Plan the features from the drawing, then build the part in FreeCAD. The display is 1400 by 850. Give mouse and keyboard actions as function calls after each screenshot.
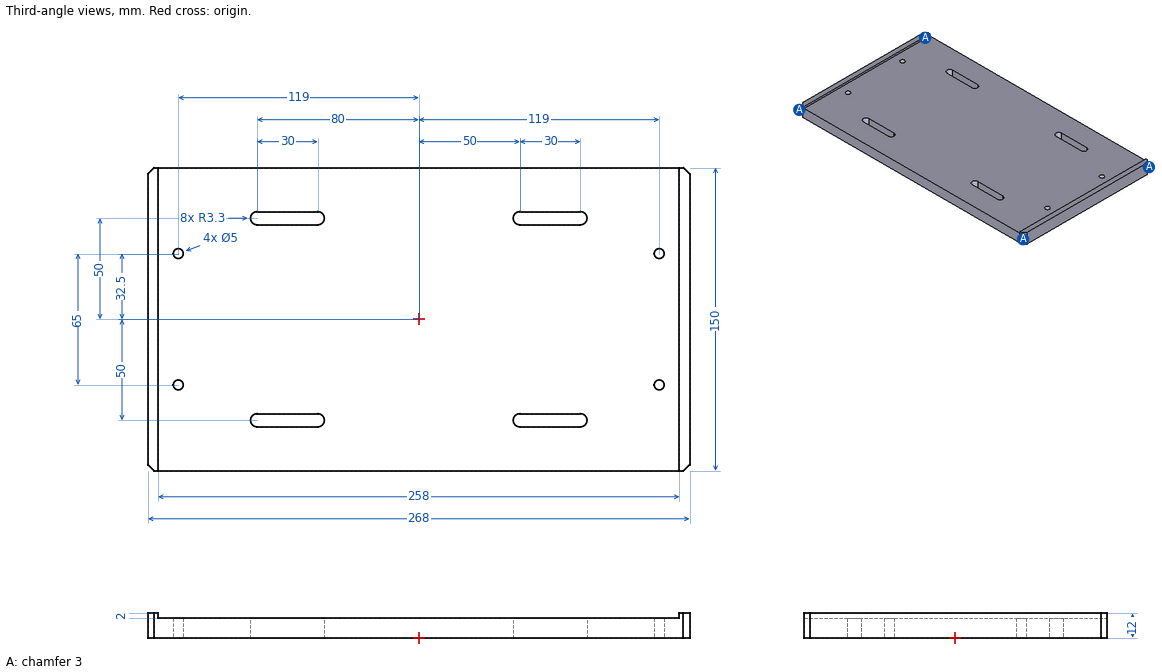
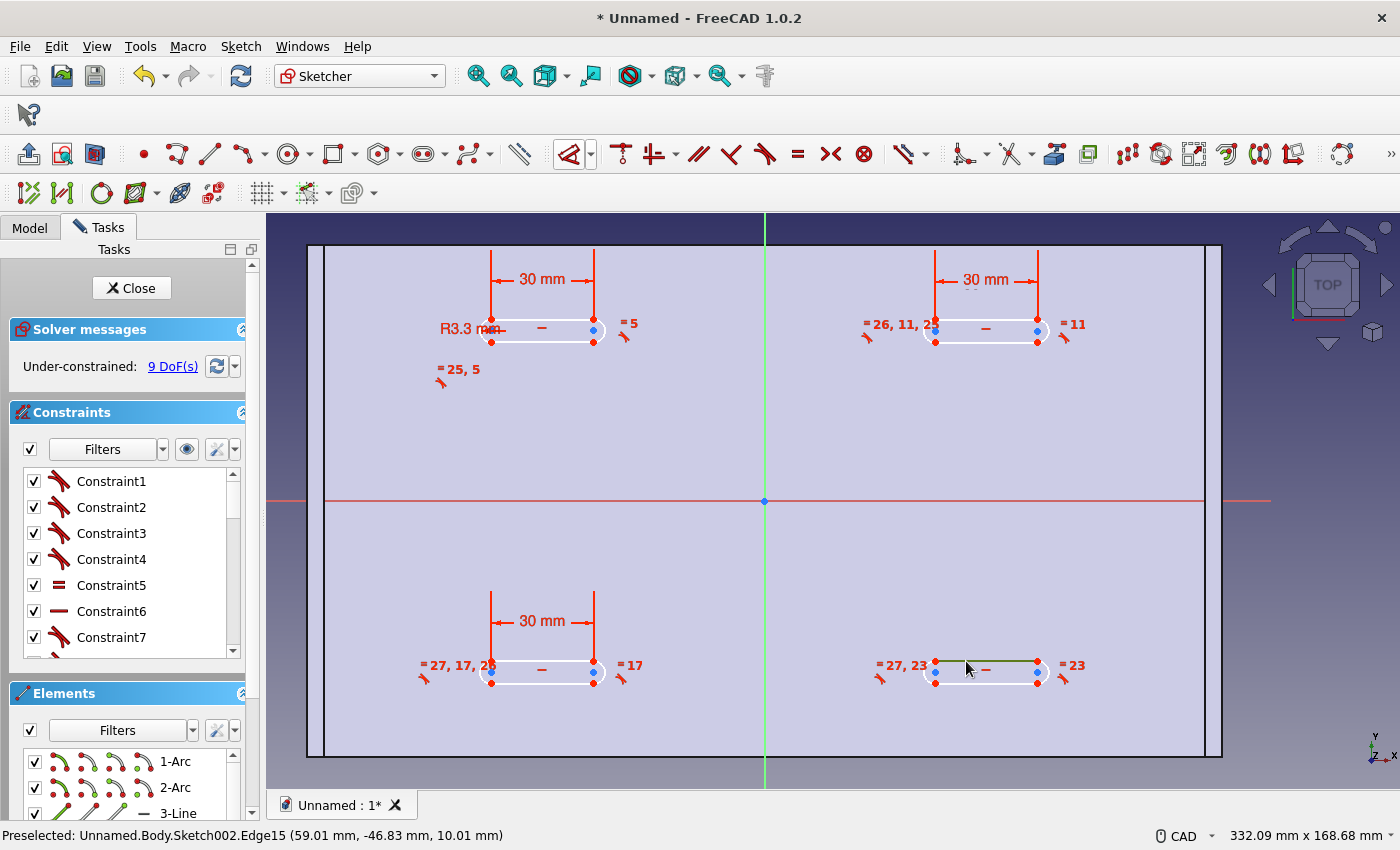
click(590, 154)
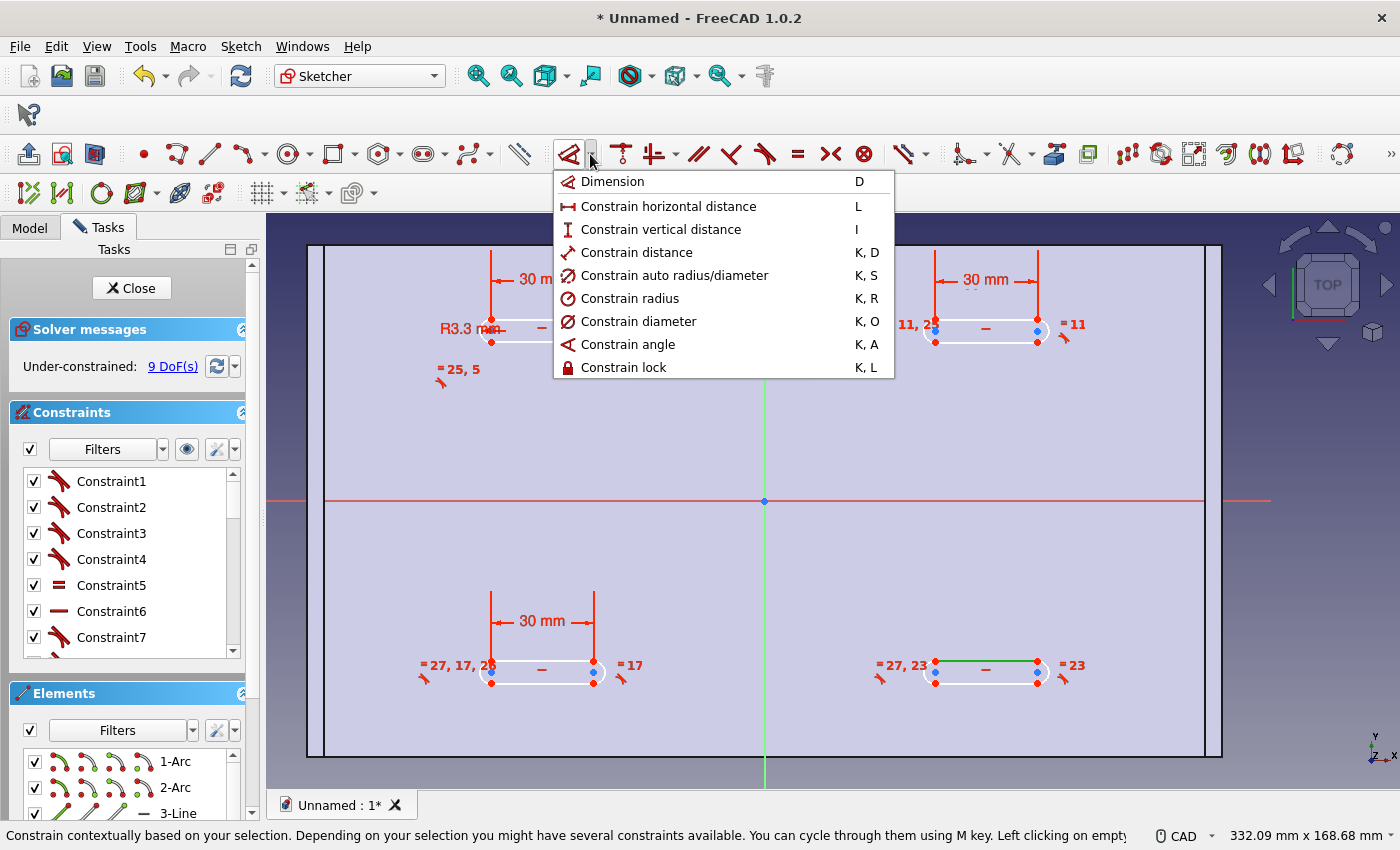
click(724, 206)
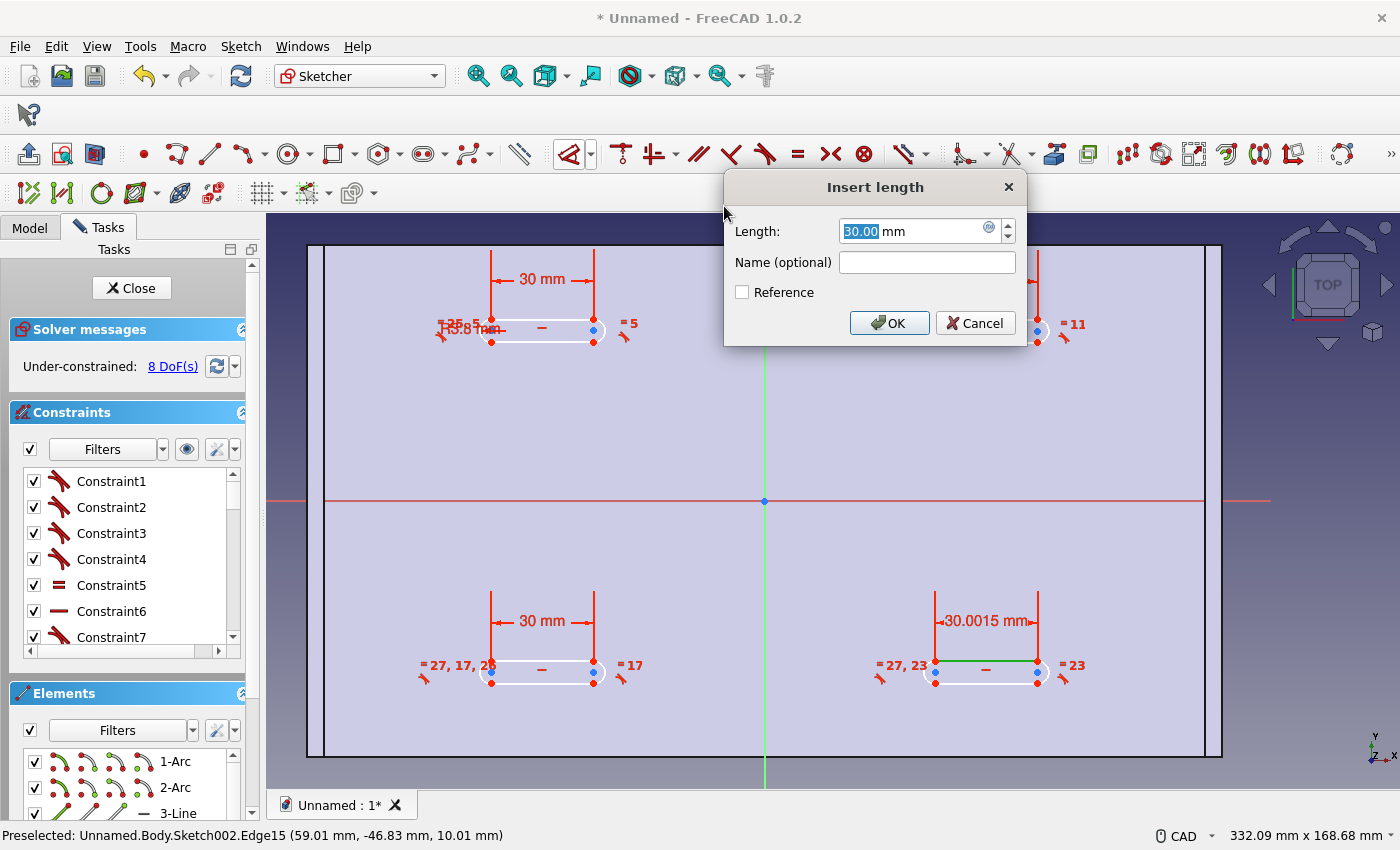
text(30)
key(Return)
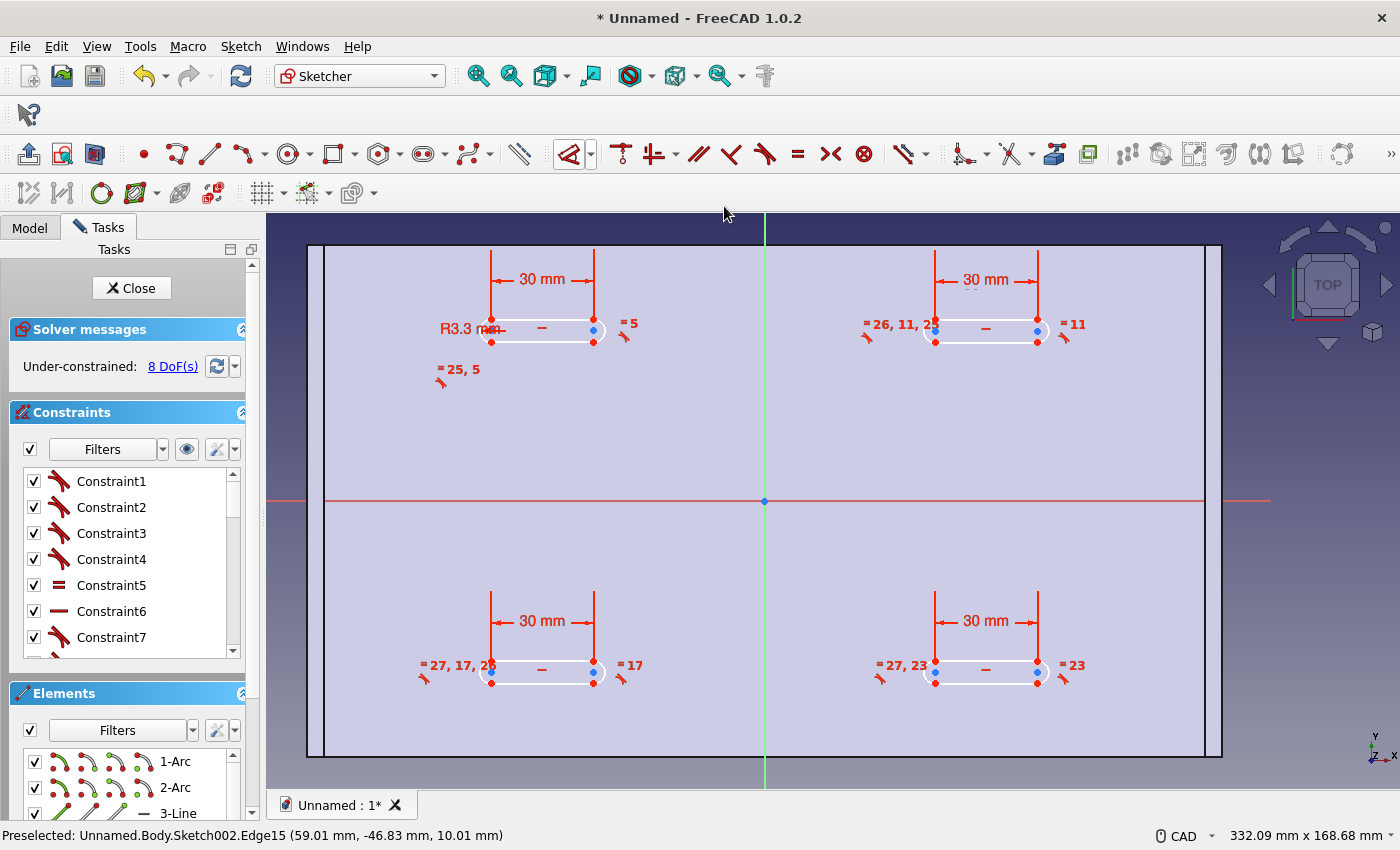
click(491, 320)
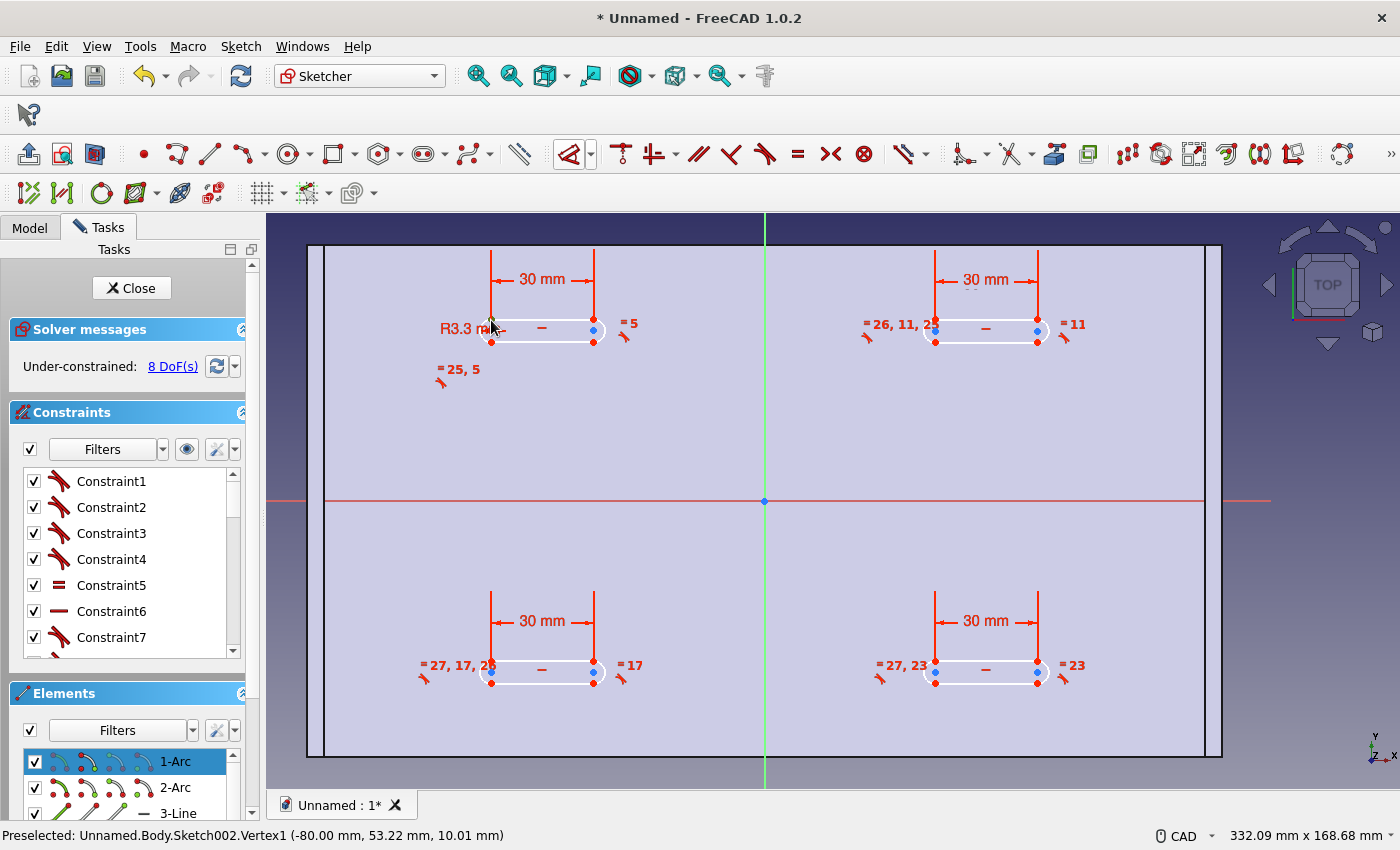
click(590, 154)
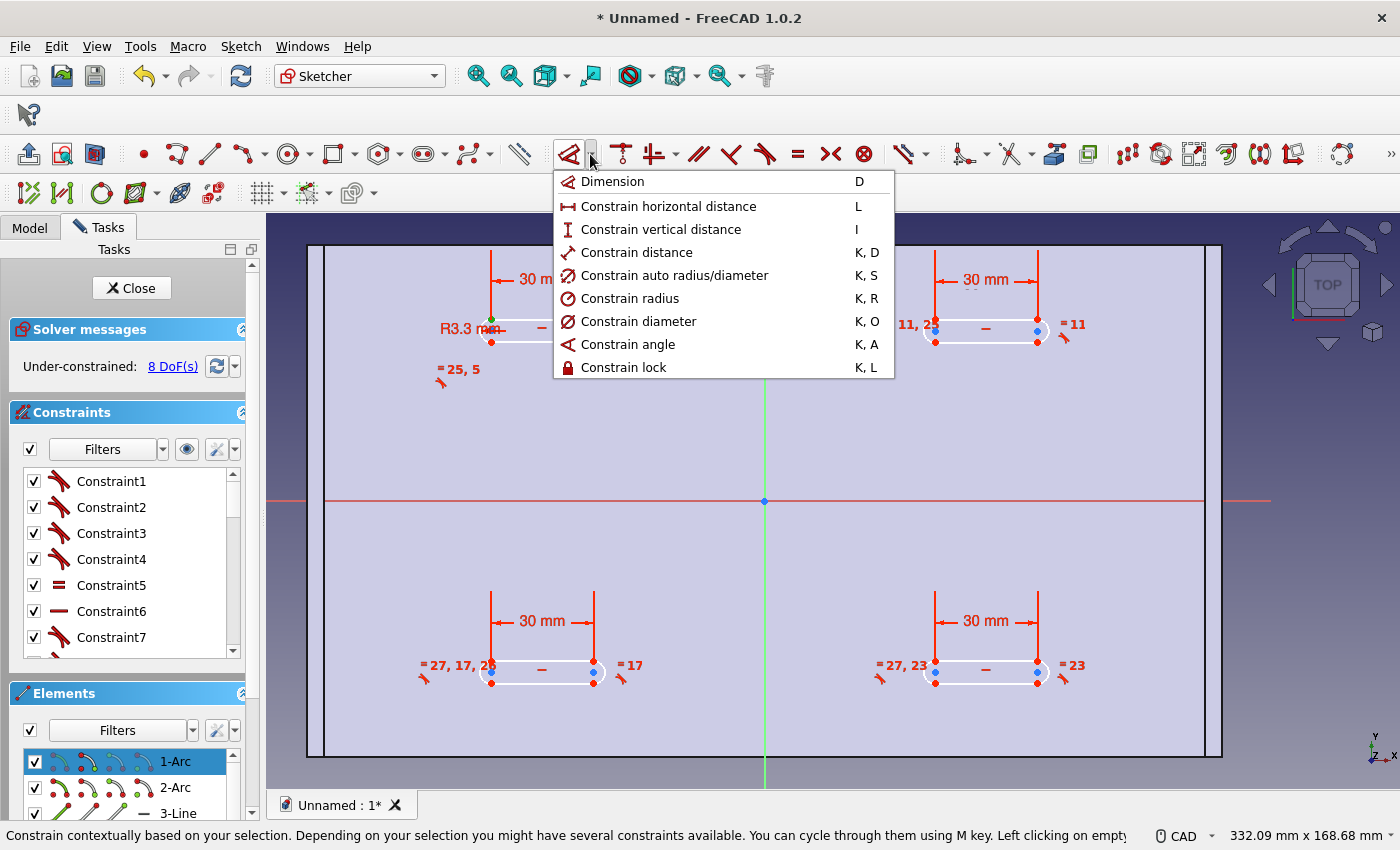
click(724, 206)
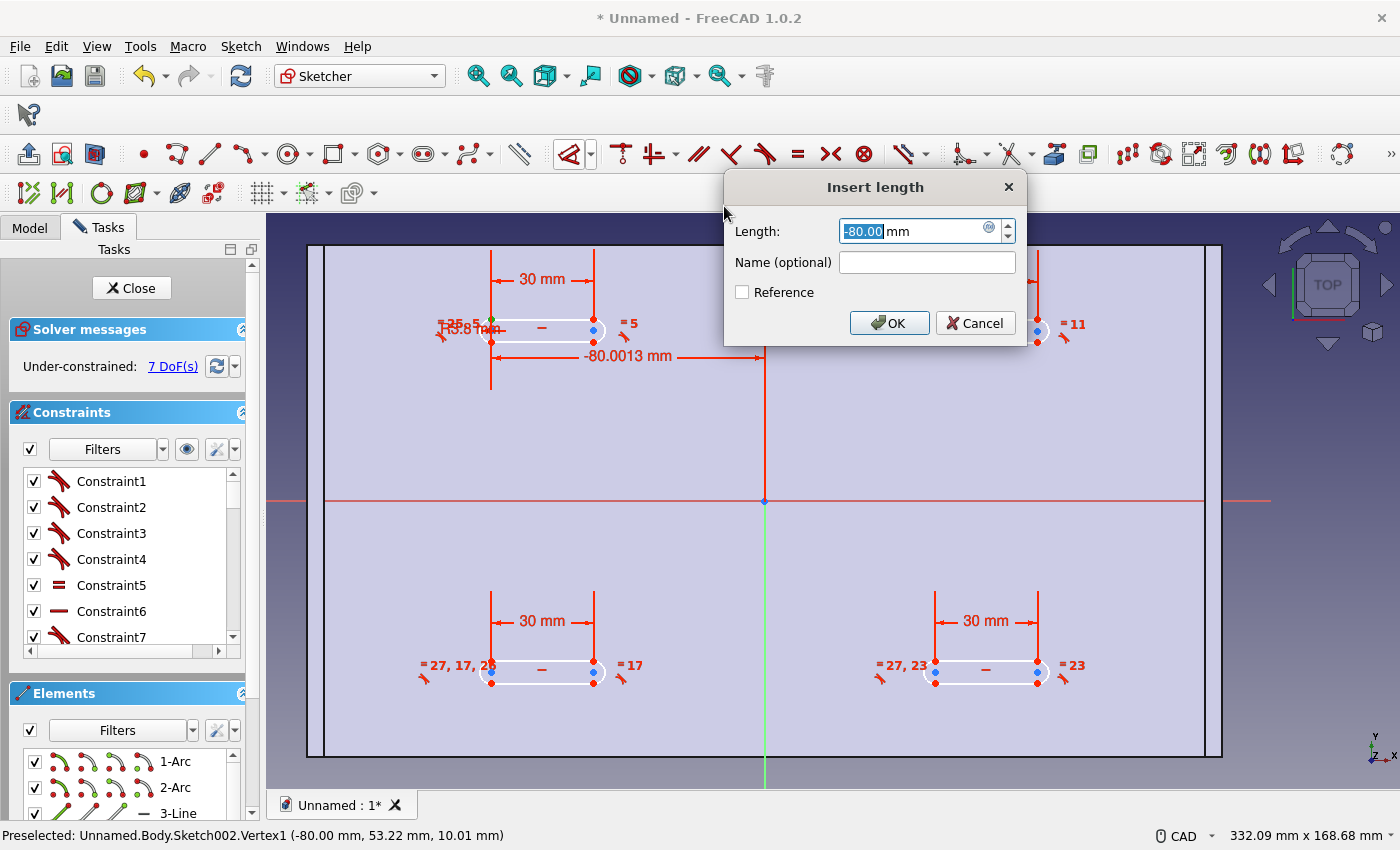
text(-80)
key(Return)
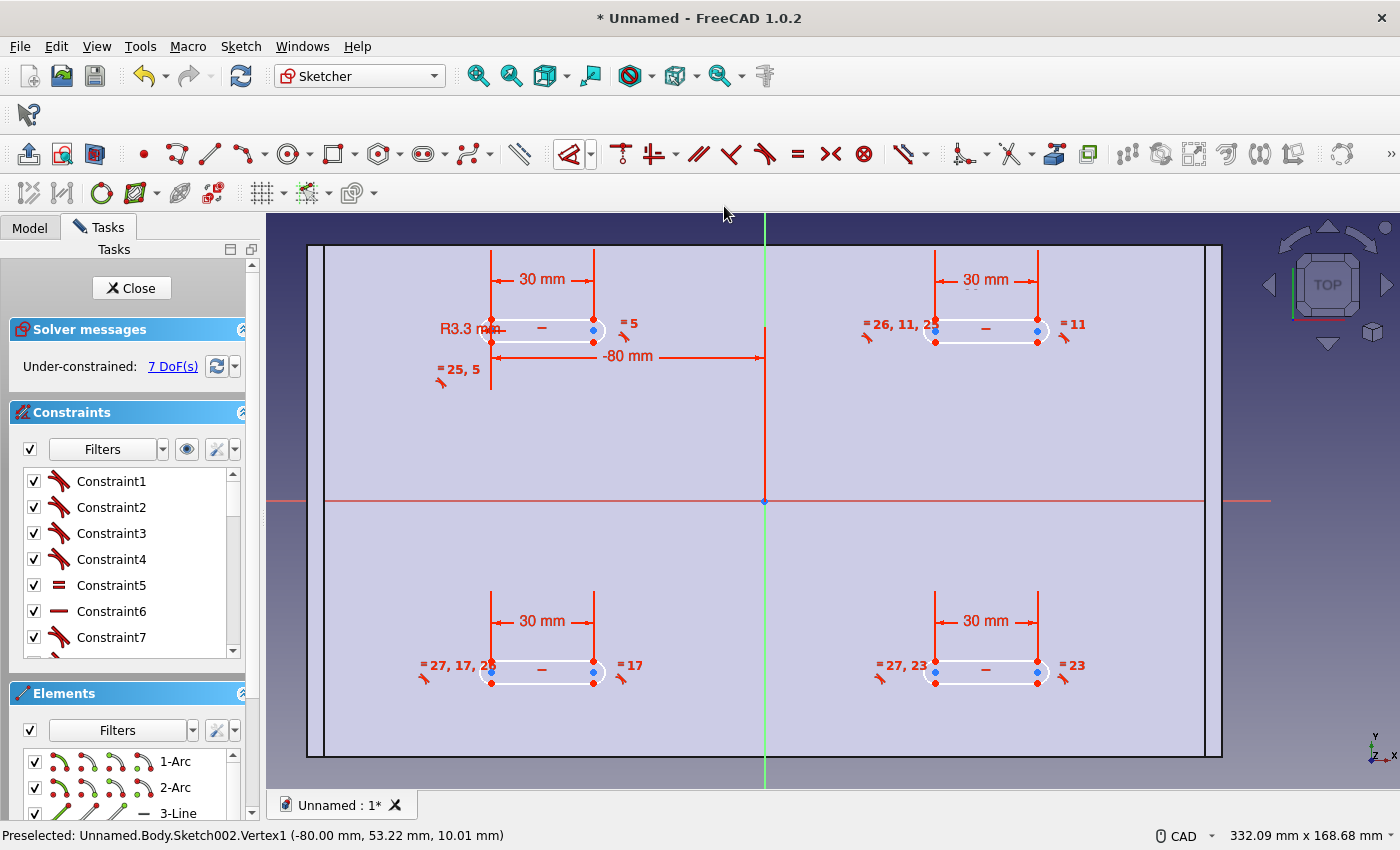
click(935, 320)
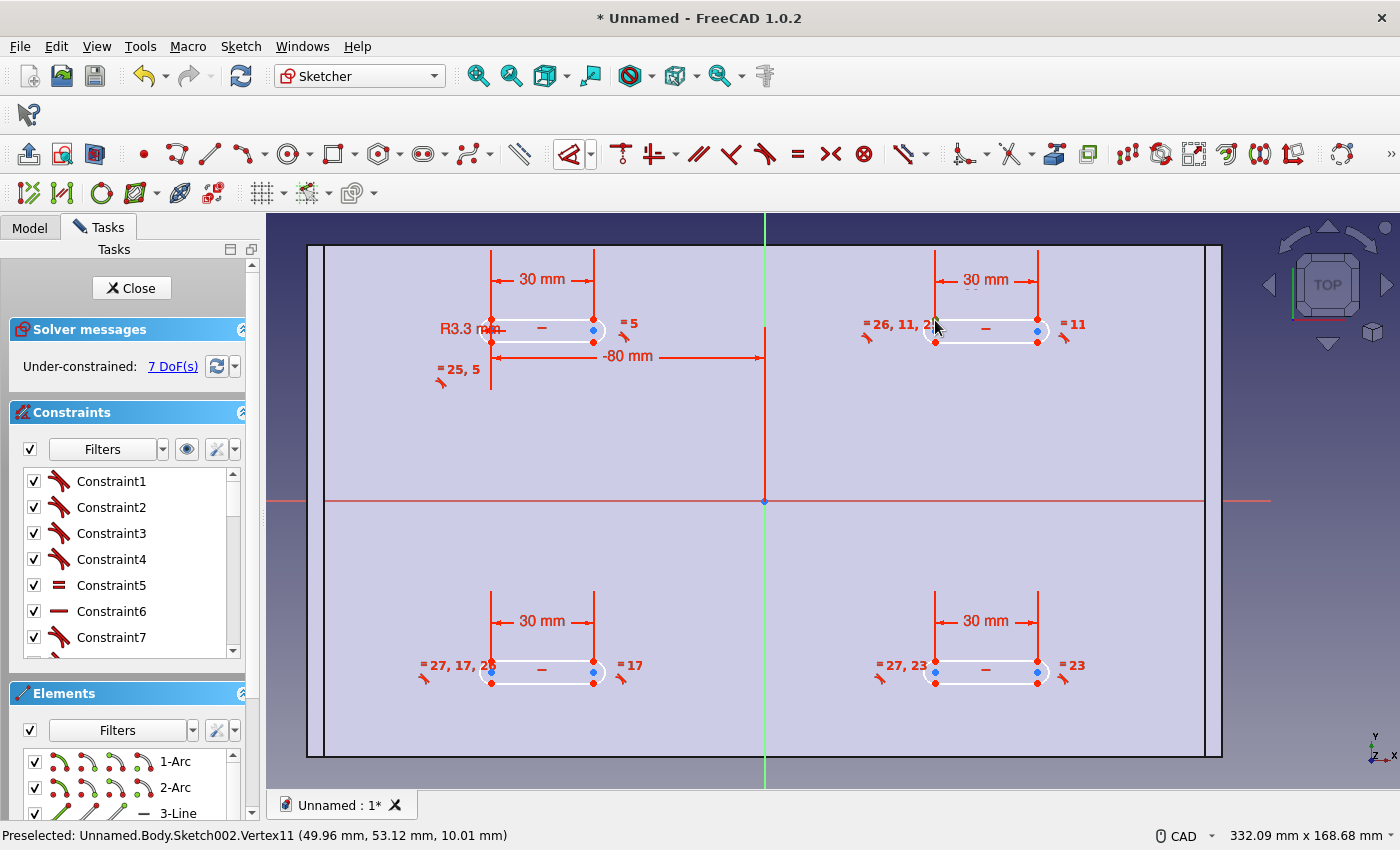
key(l)